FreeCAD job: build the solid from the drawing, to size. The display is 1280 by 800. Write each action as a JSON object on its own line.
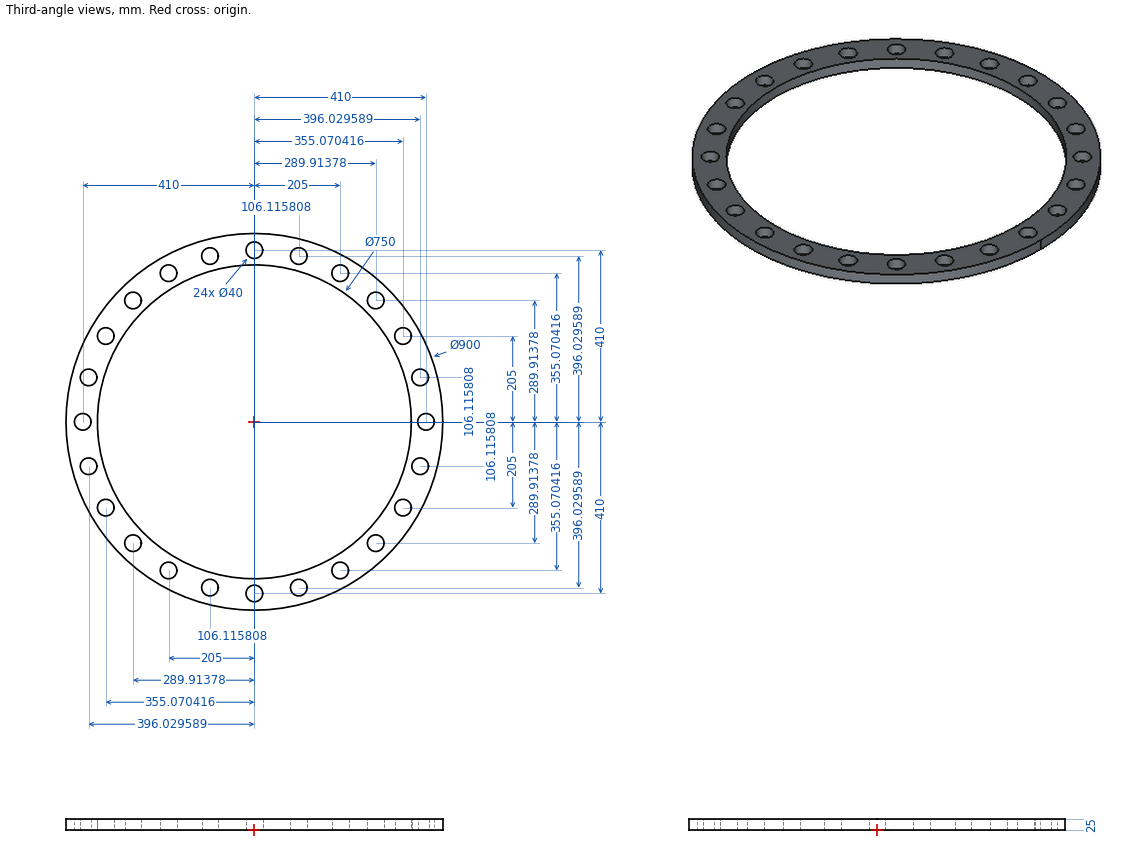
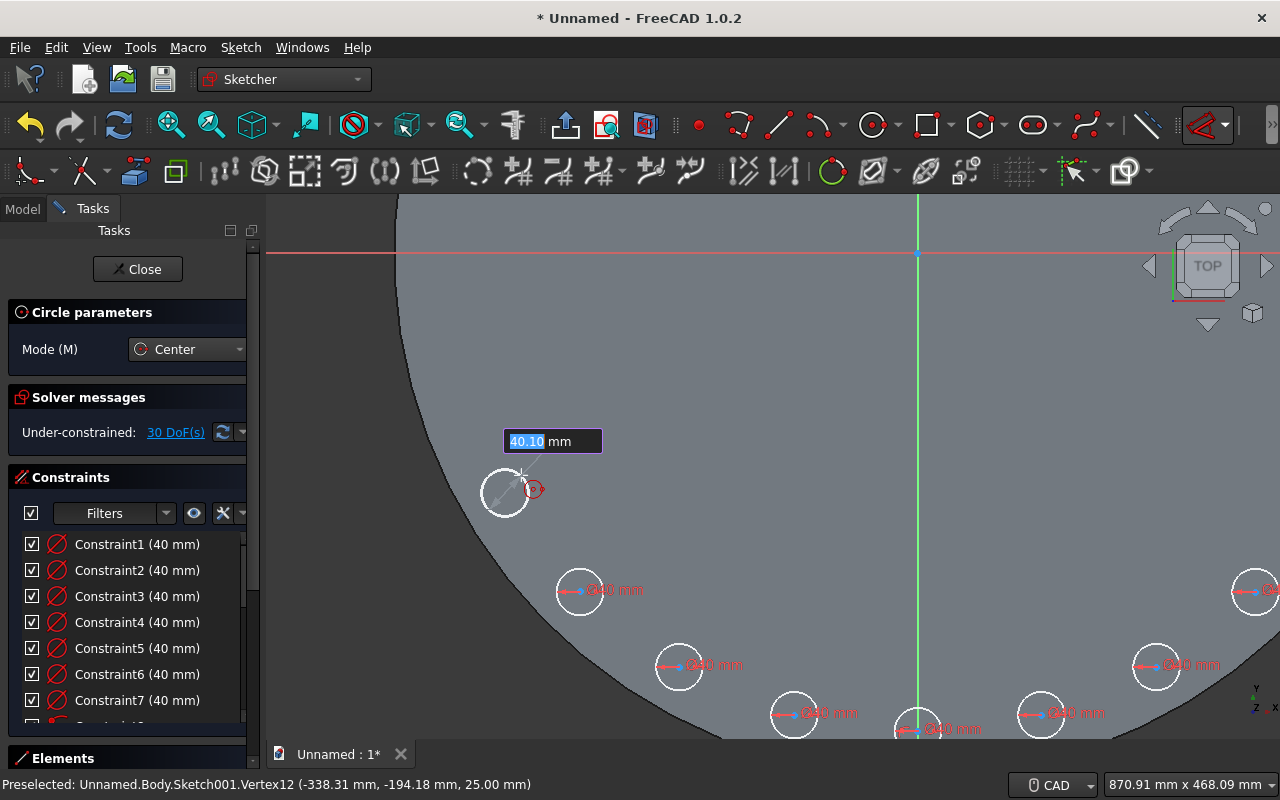
{"action": "type", "text": "40"}
{"action": "key", "text": "Return"}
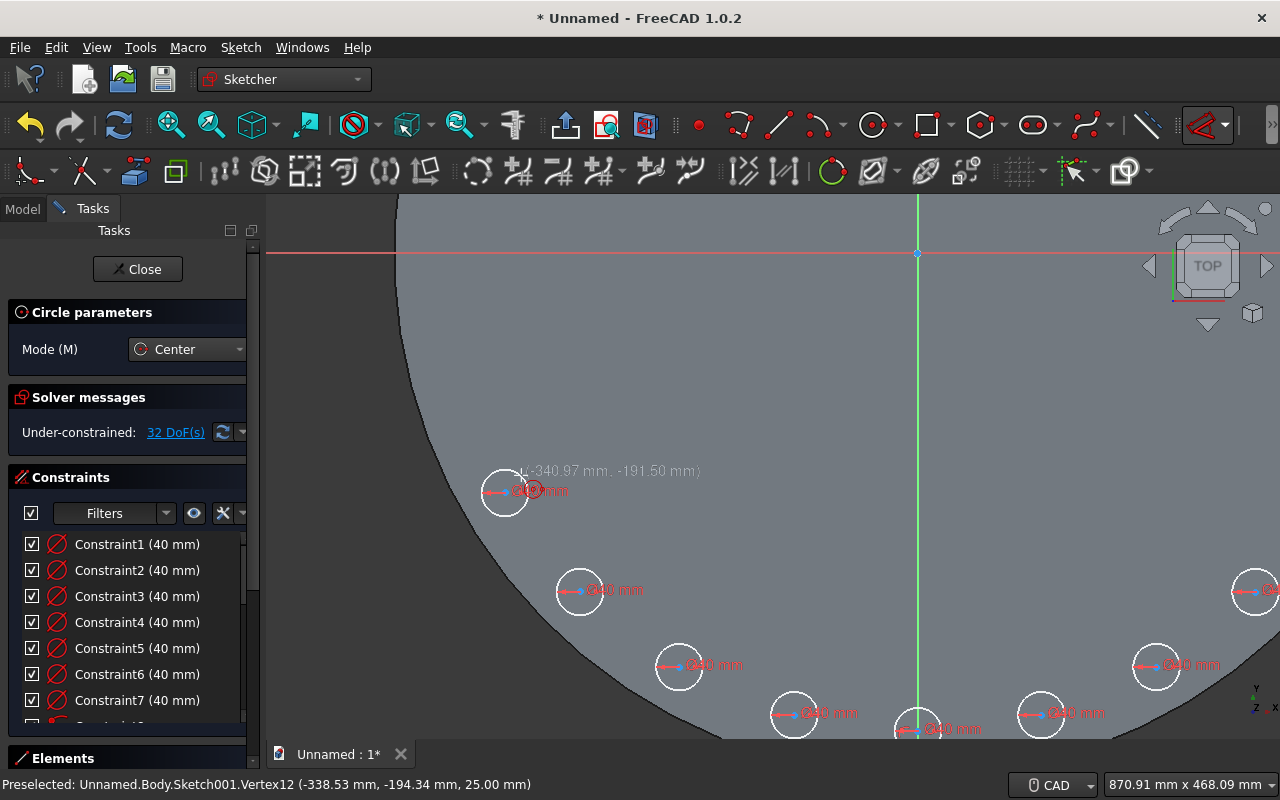
{"action": "left_click", "coordinate": [457, 377]}
{"action": "mouse_move", "coordinate": [473, 360]}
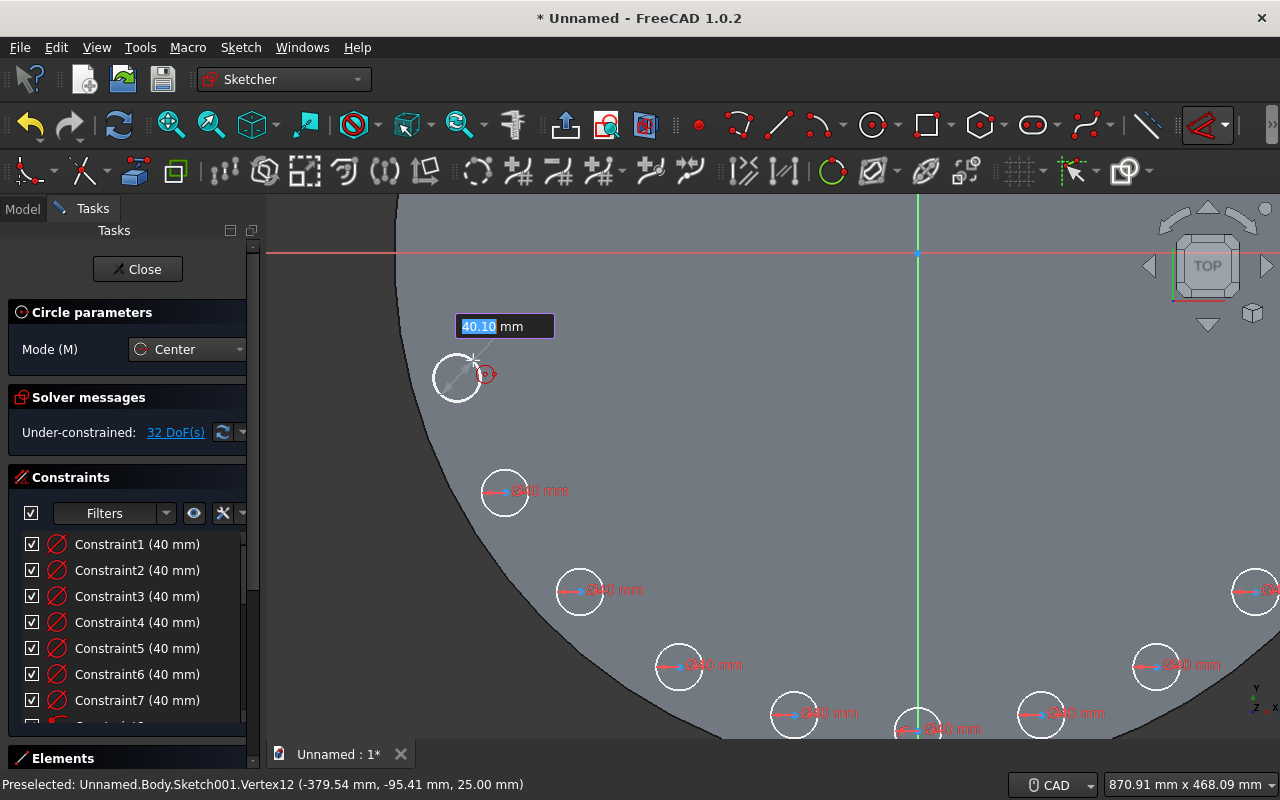
{"action": "type", "text": "40"}
{"action": "key", "text": "Return"}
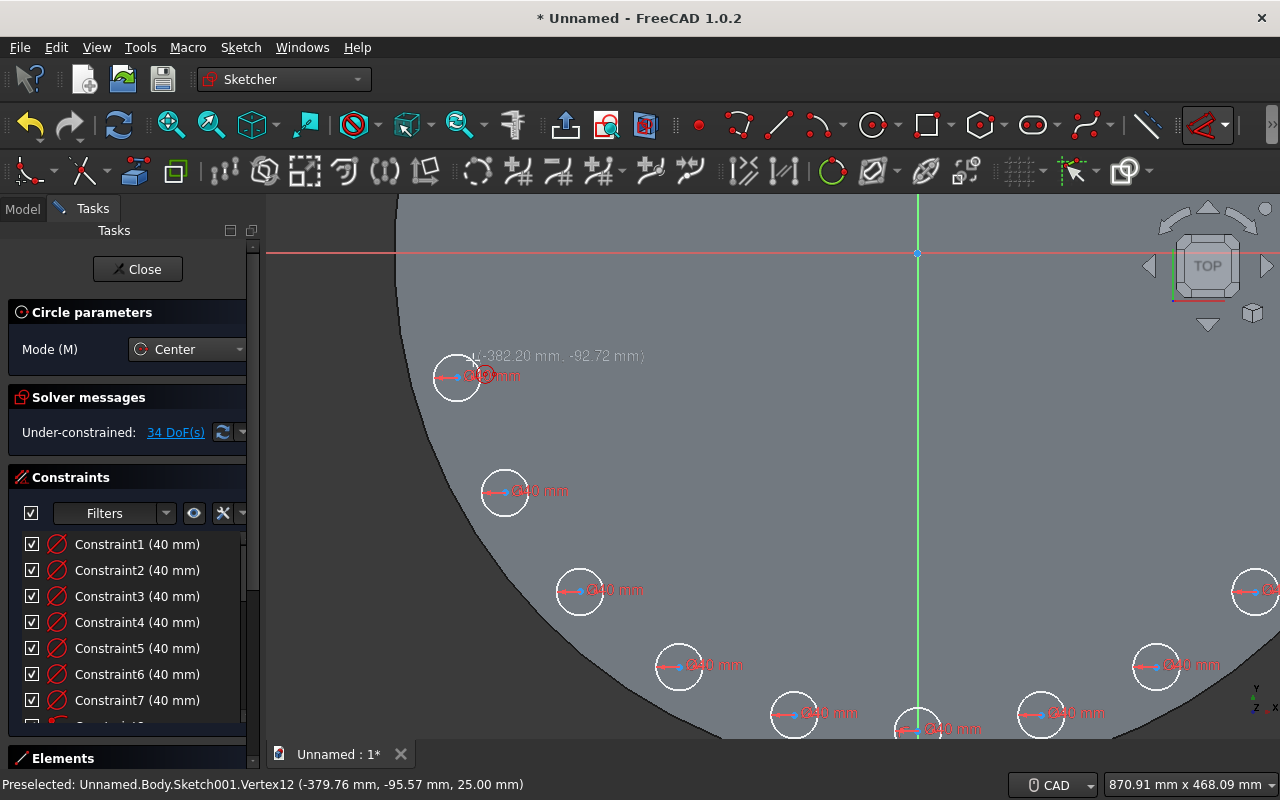
{"action": "left_click", "coordinate": [441, 253]}
{"action": "mouse_move", "coordinate": [457, 237]}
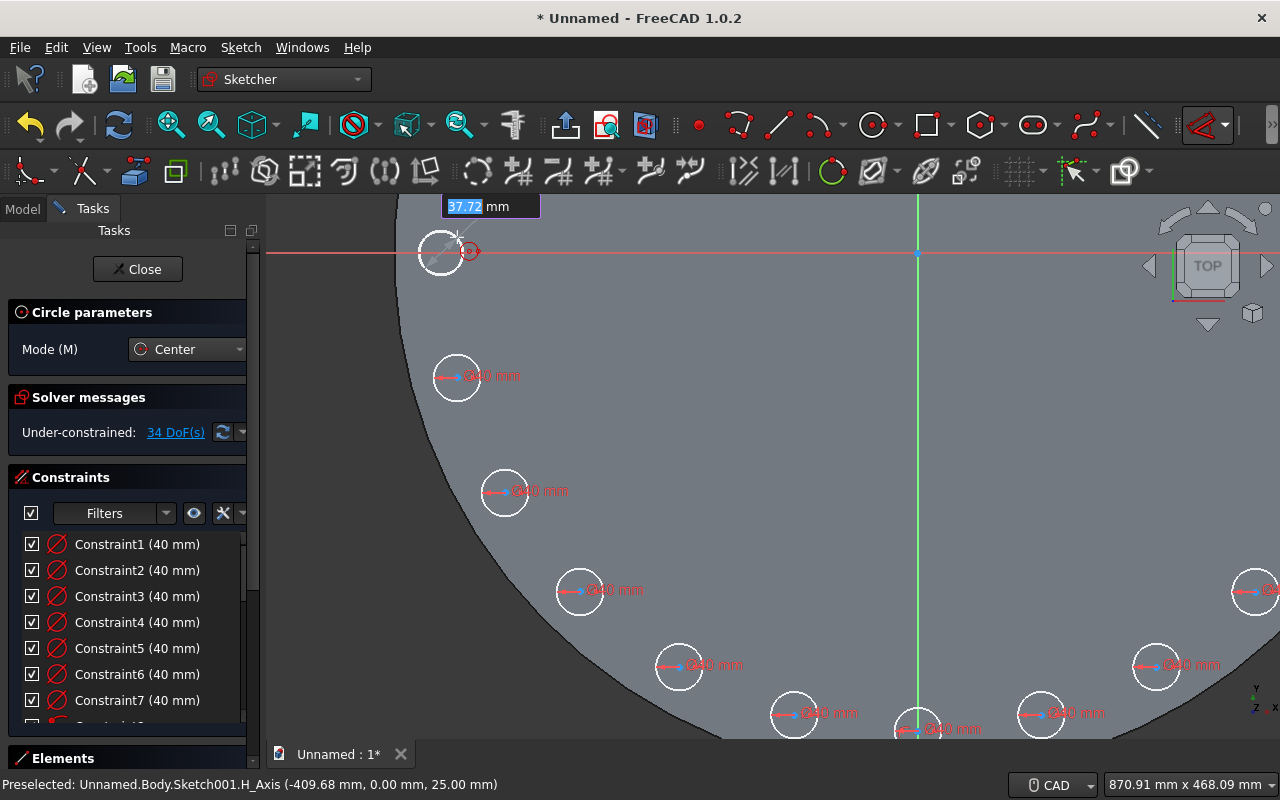
{"action": "type", "text": "40"}
{"action": "key", "text": "Return"}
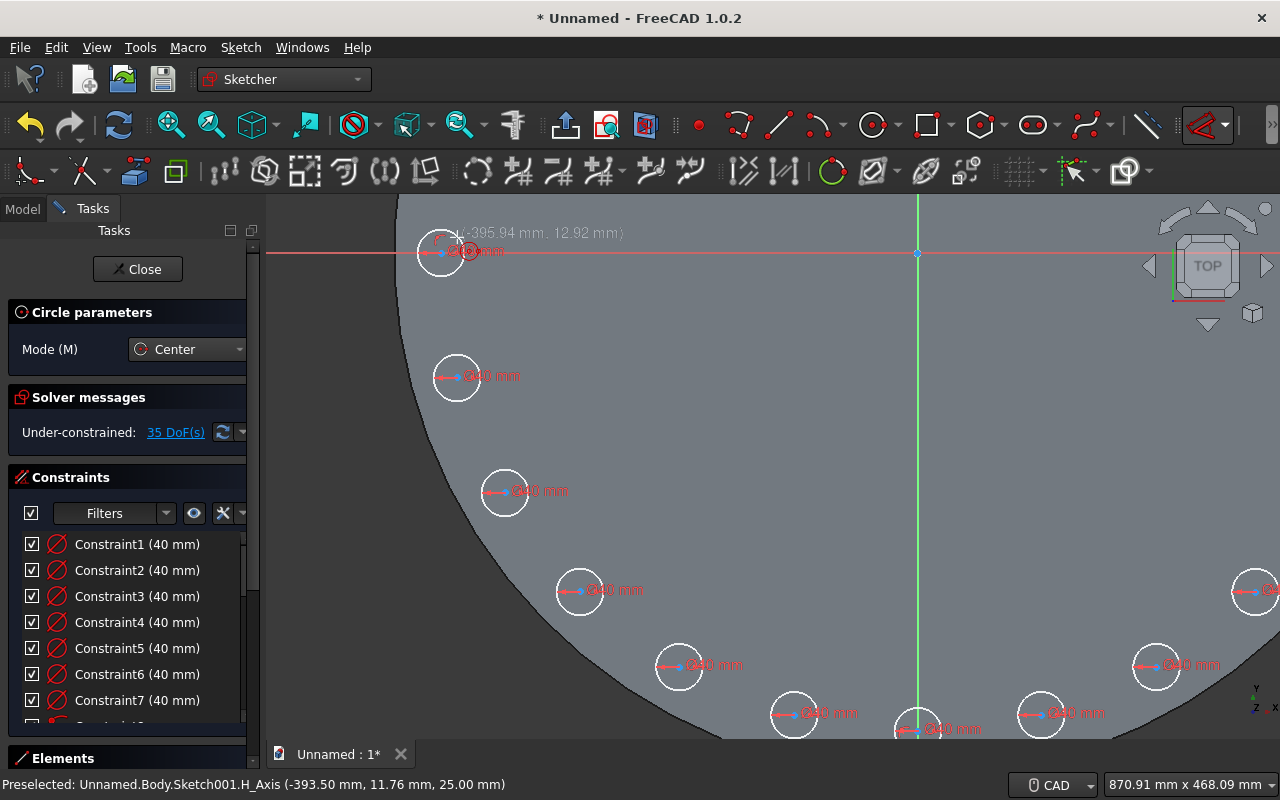
{"action": "scroll", "coordinate": [580, 591], "scroll_direction": "down", "scroll_amount": 5}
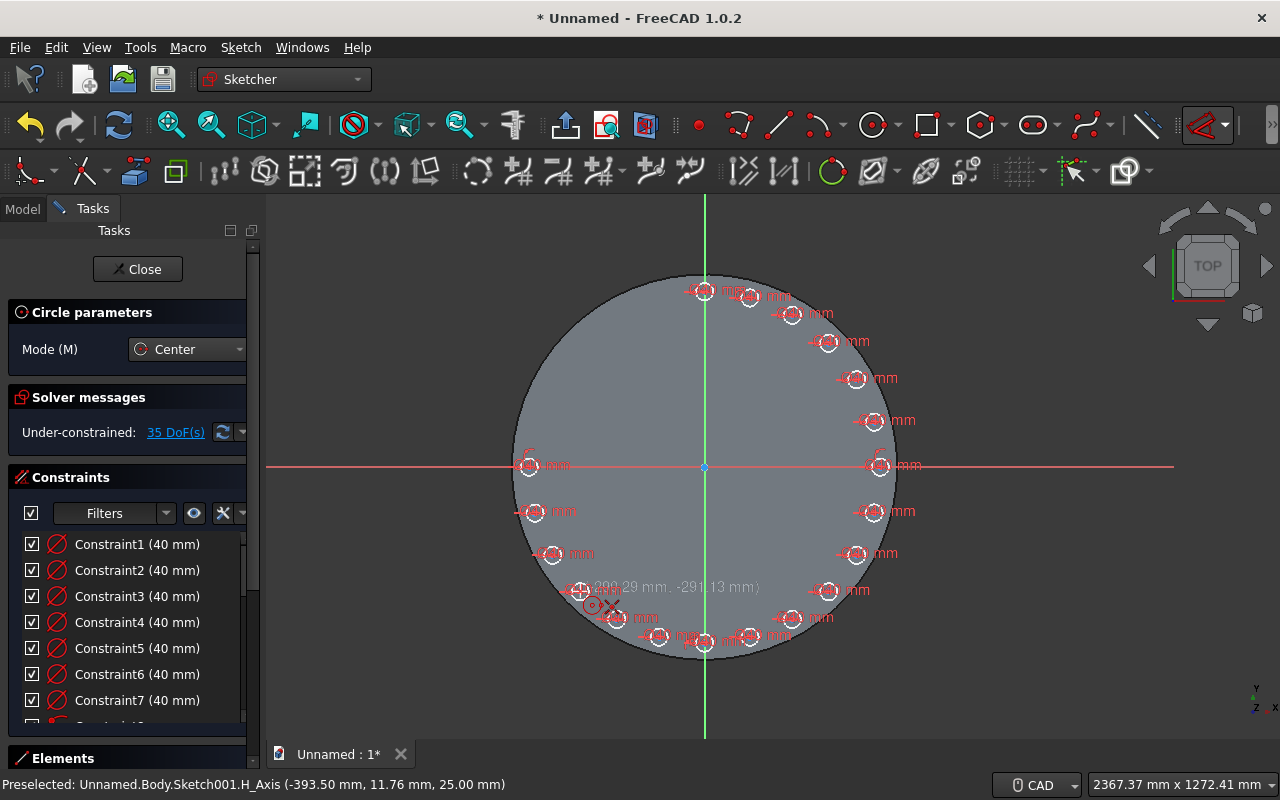
{"action": "scroll", "coordinate": [535, 422], "scroll_direction": "up", "scroll_amount": 5}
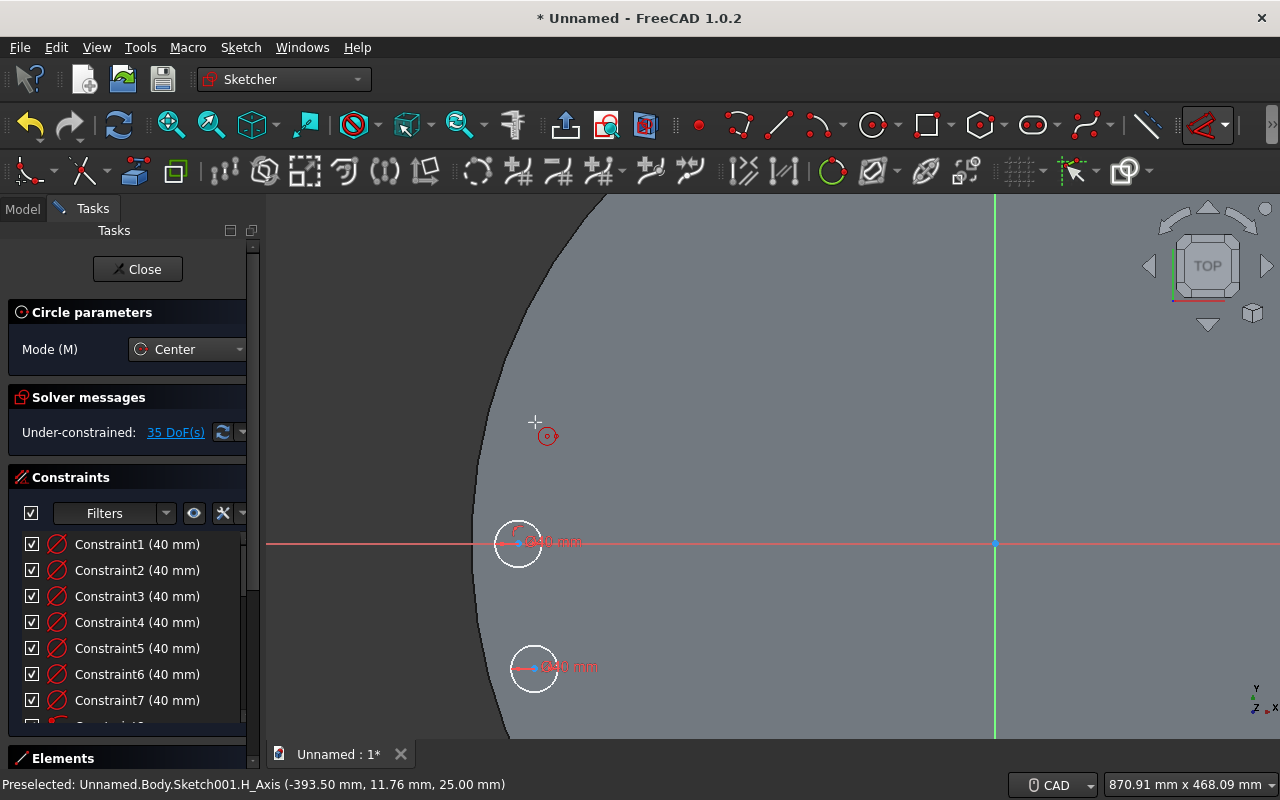
{"action": "left_click", "coordinate": [534, 420]}
{"action": "mouse_move", "coordinate": [551, 404]}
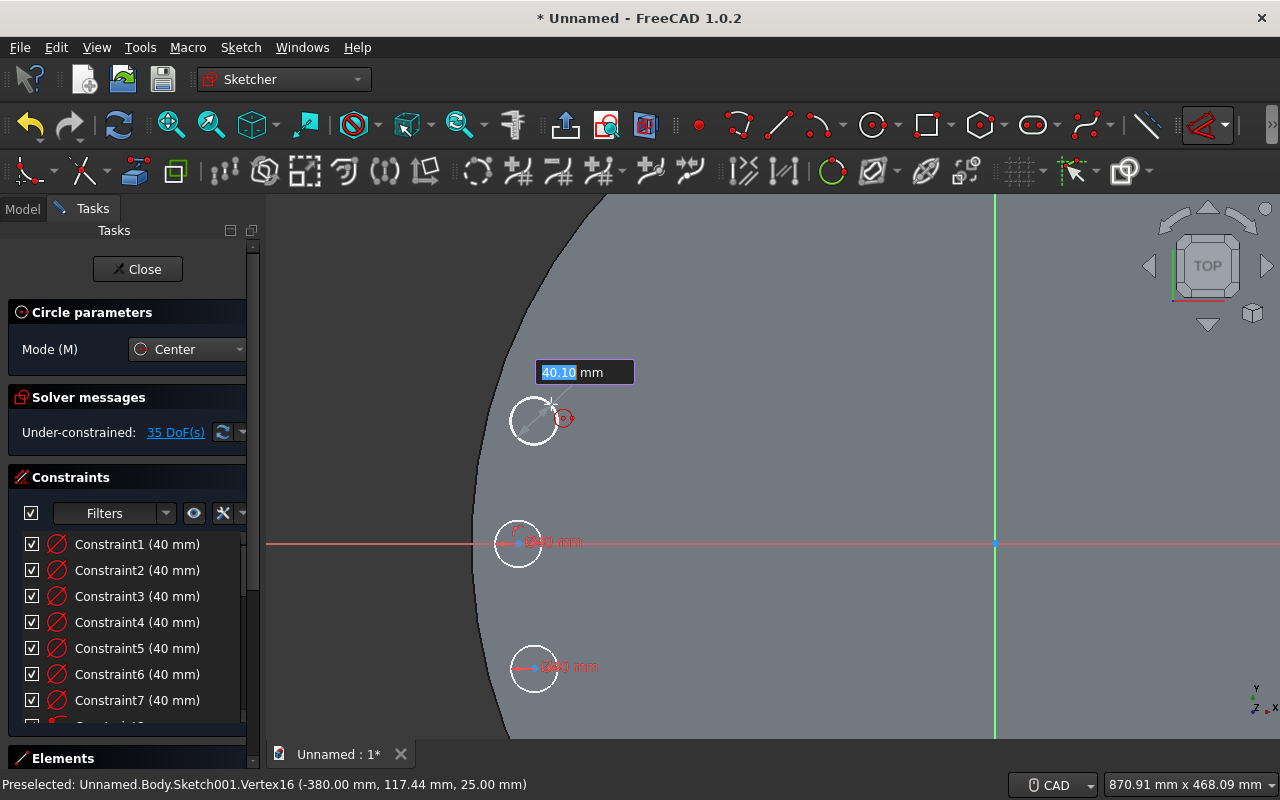
{"action": "type", "text": "40"}
{"action": "key", "text": "Return"}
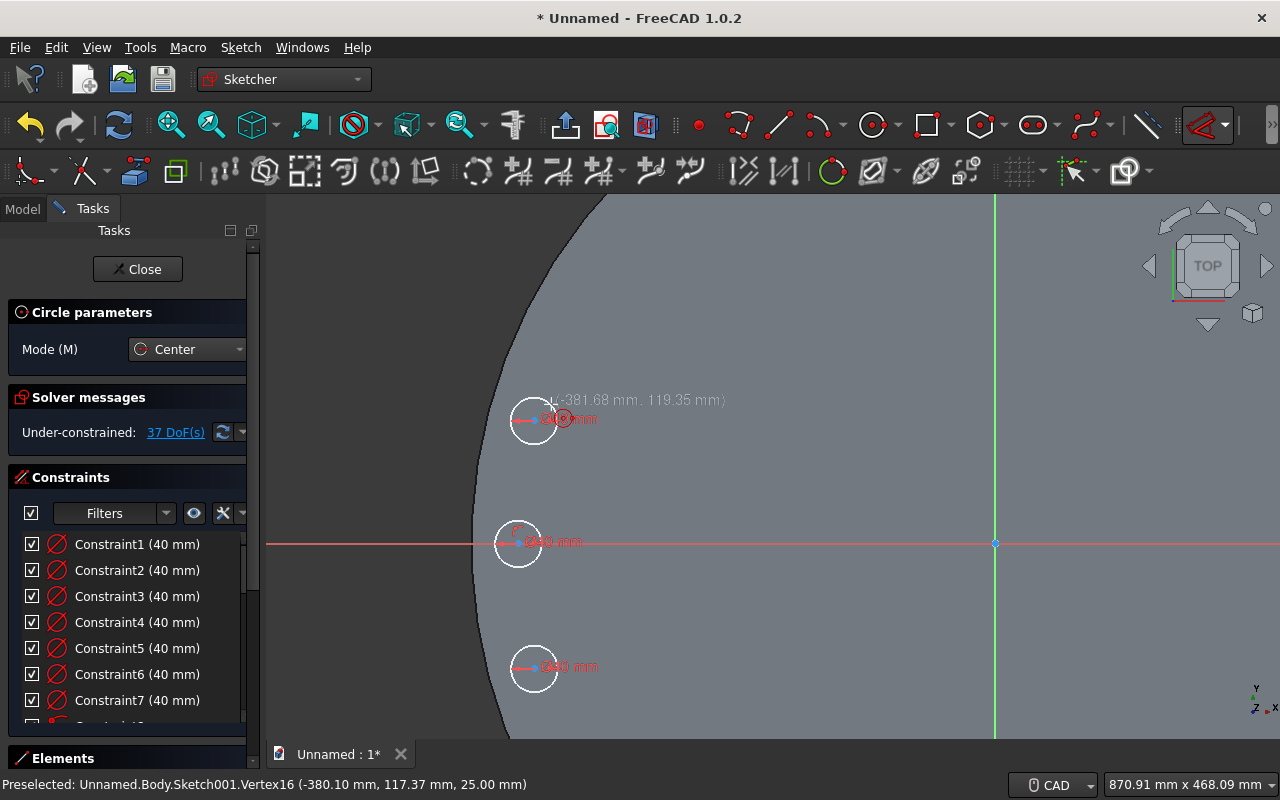
{"action": "left_click", "coordinate": [582, 305]}
{"action": "mouse_move", "coordinate": [598, 289]}